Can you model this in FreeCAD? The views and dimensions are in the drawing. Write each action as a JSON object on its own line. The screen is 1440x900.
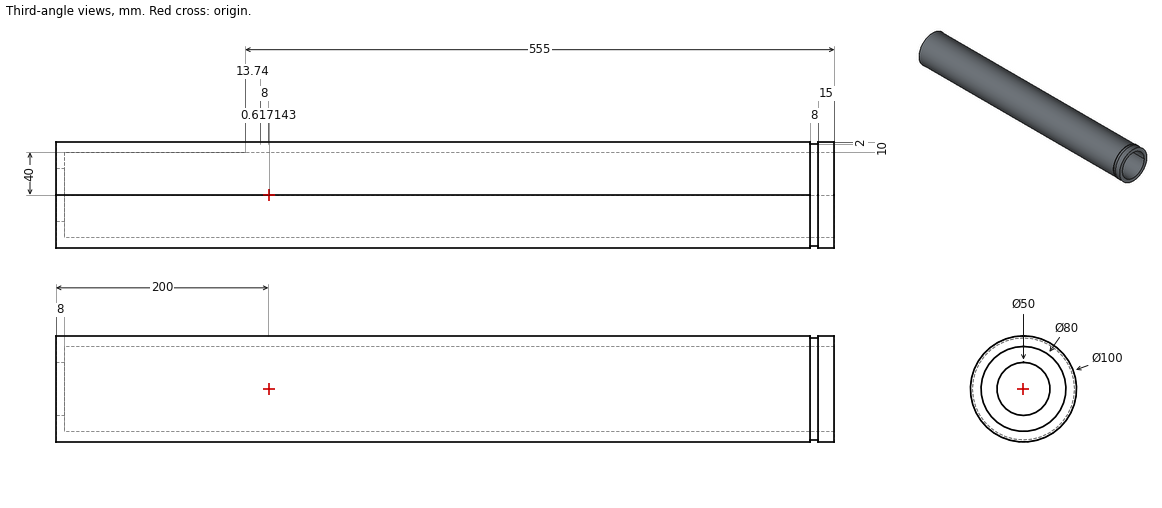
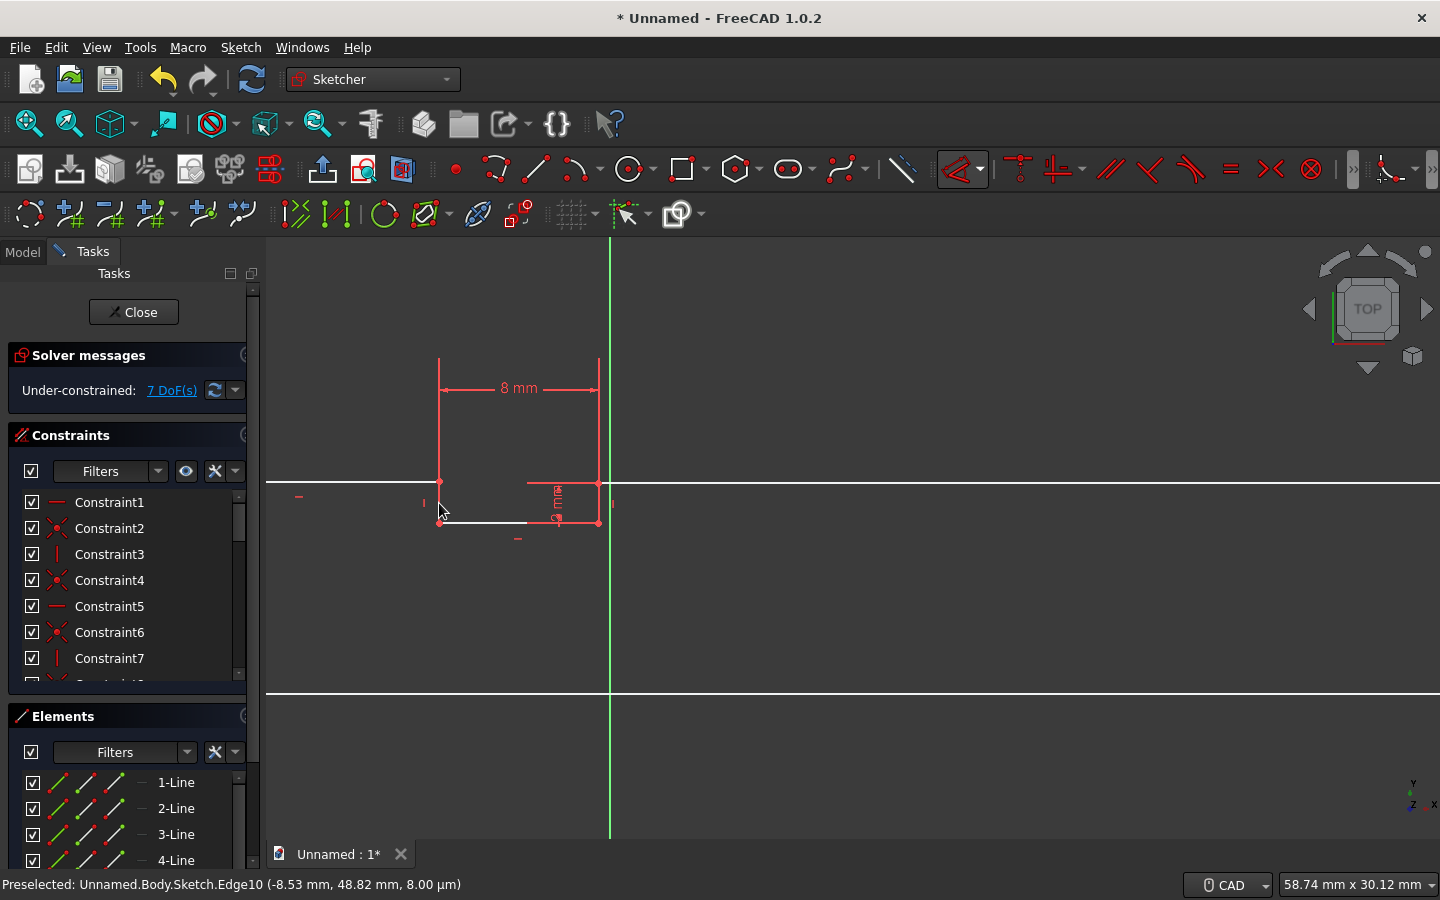
{"action": "key", "text": "i"}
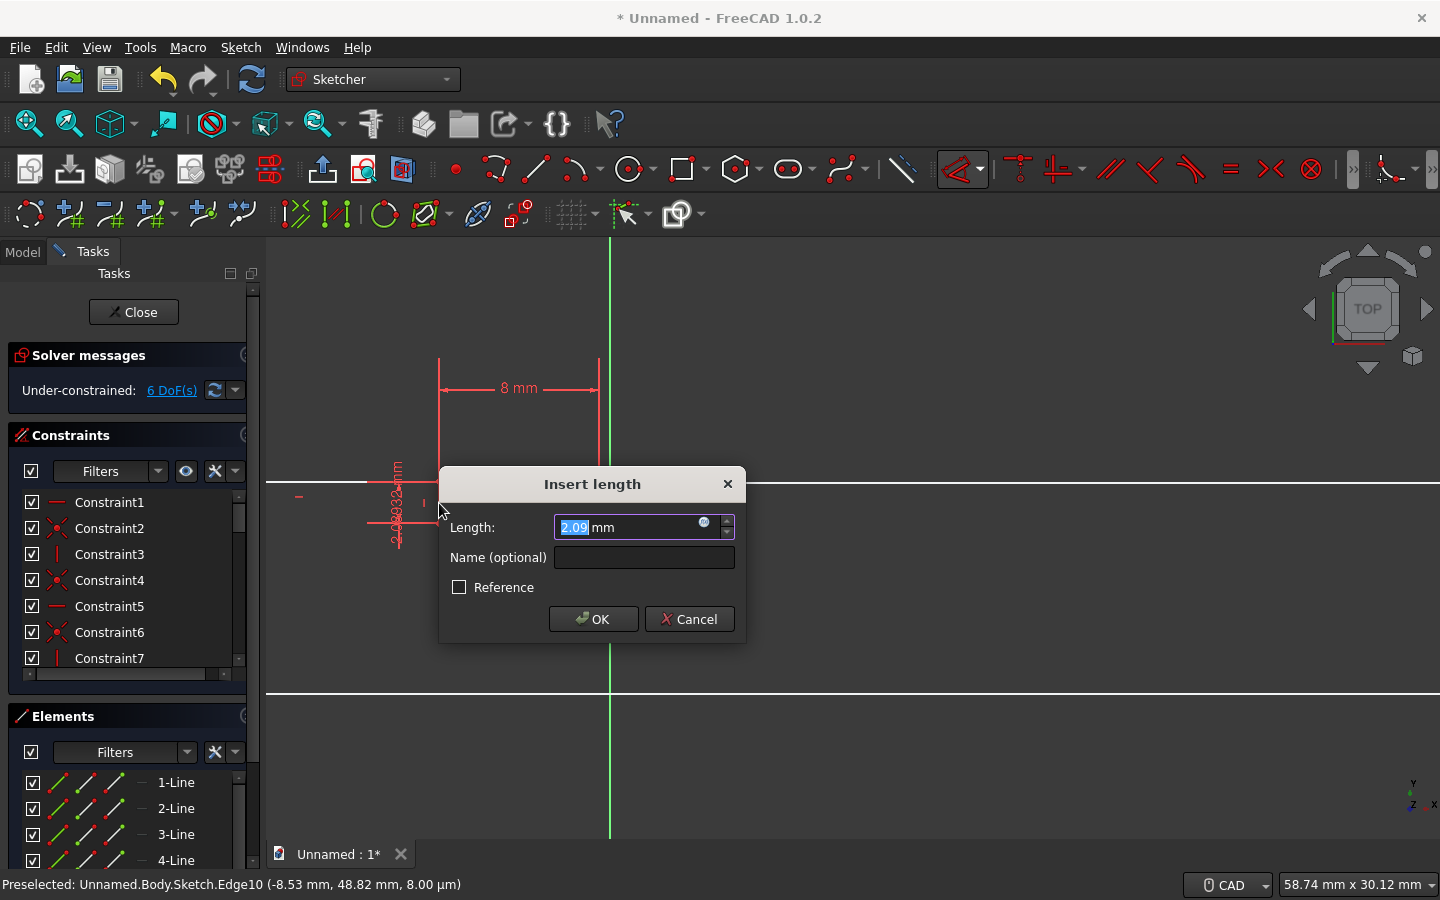
{"action": "type", "text": "2"}
{"action": "key", "text": "Return"}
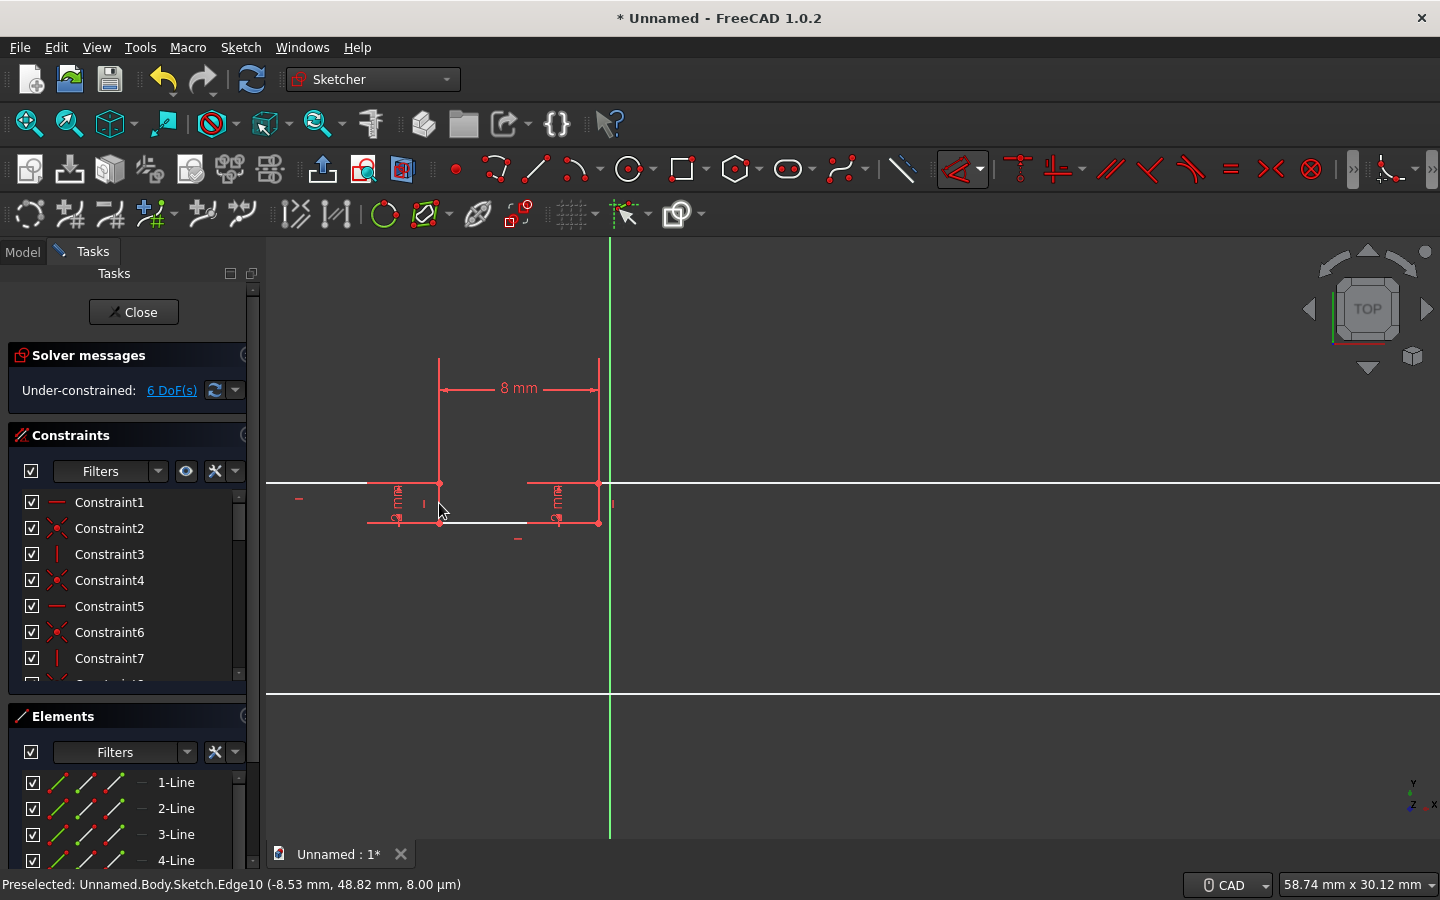
{"action": "scroll", "coordinate": [466, 509], "scroll_direction": "down", "scroll_amount": 14}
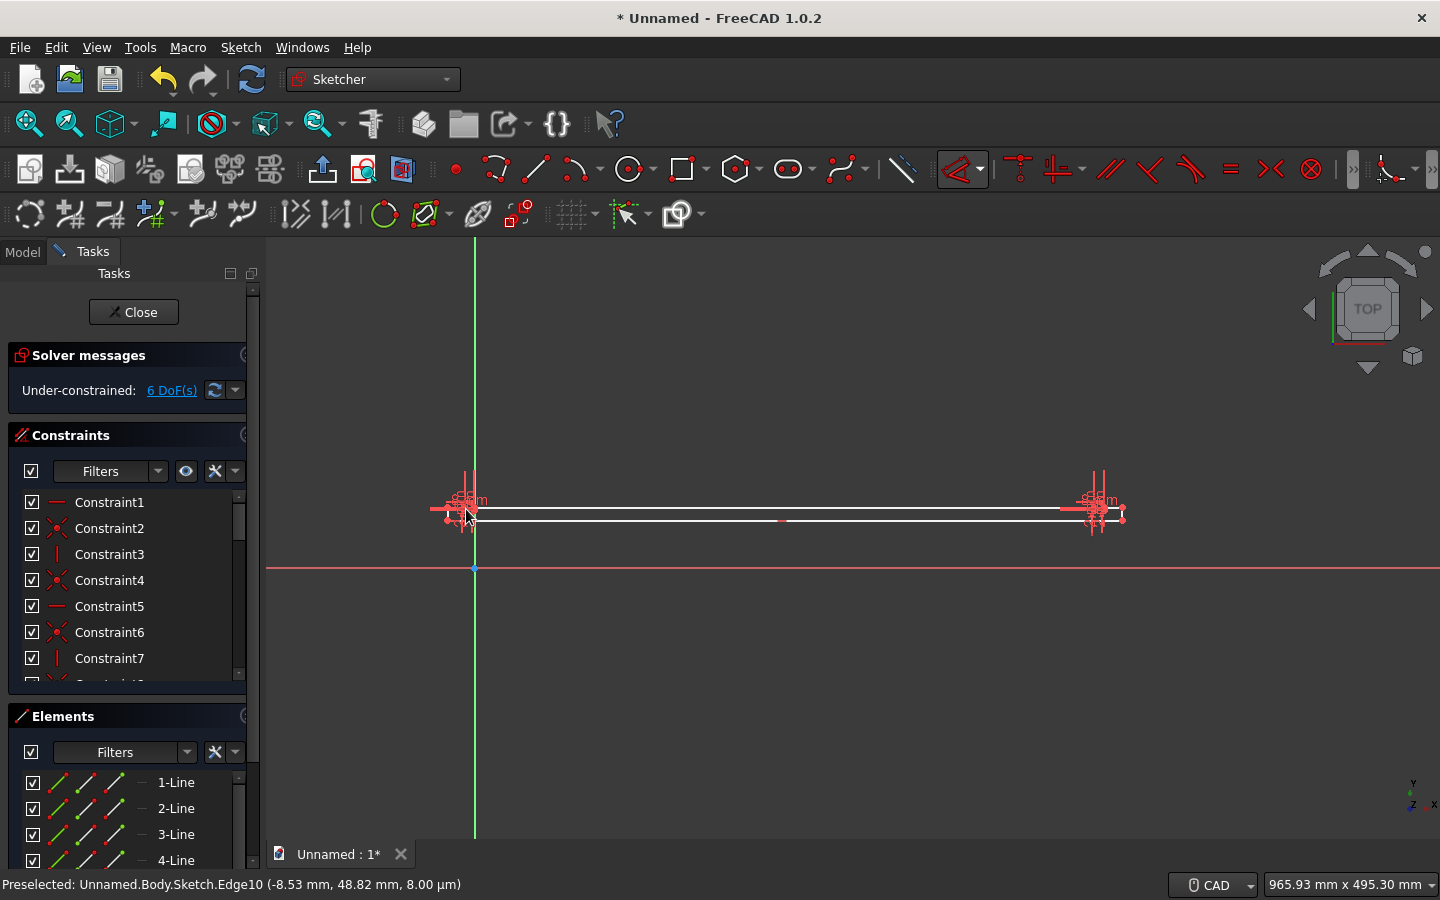
{"action": "scroll", "coordinate": [1122, 517], "scroll_direction": "up", "scroll_amount": 7}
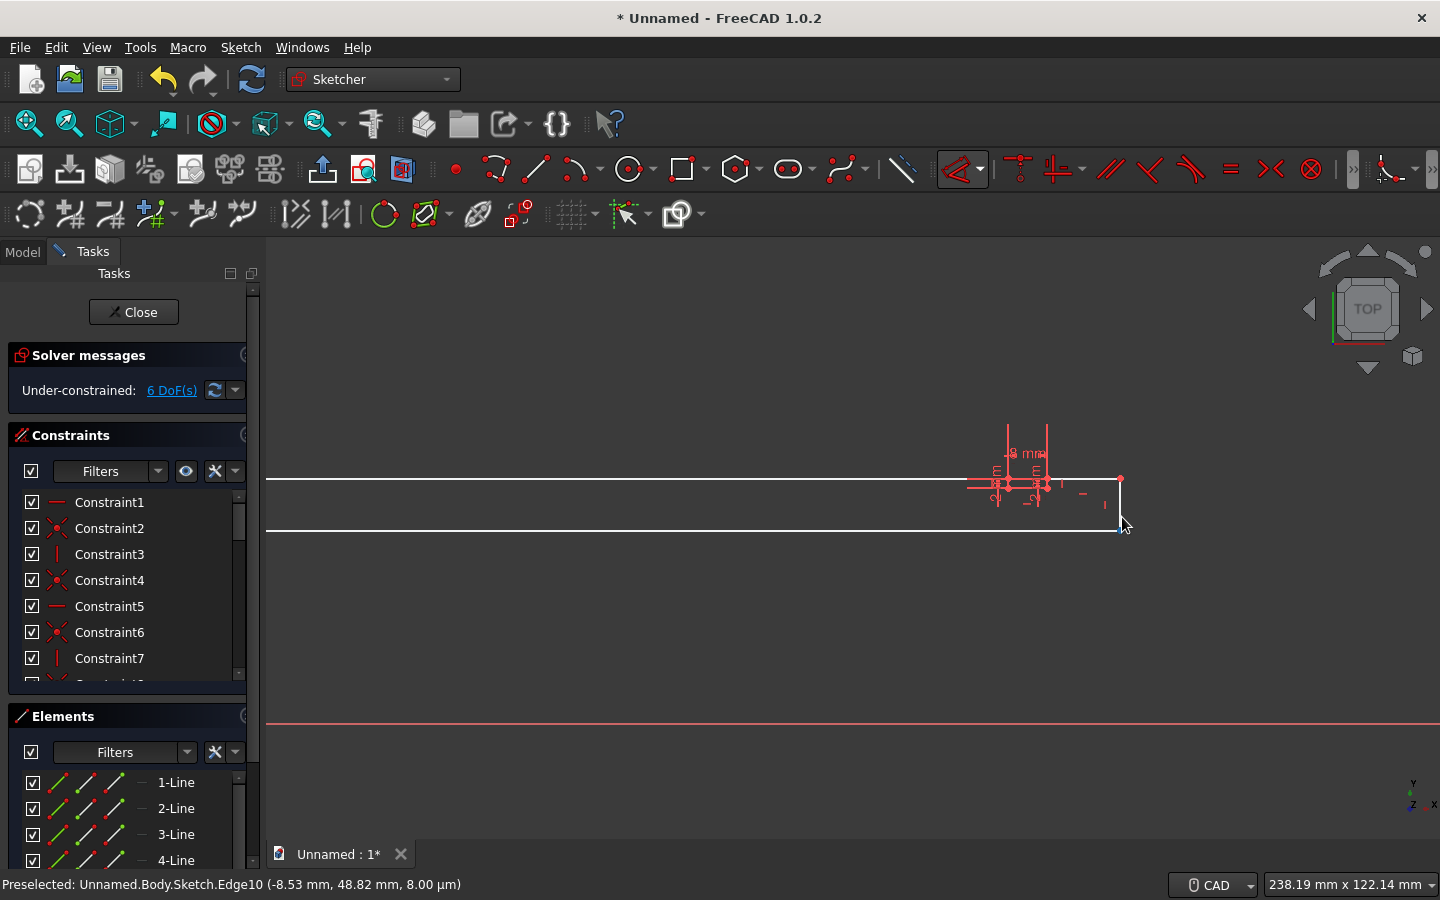
{"action": "left_click", "coordinate": [1120, 515]}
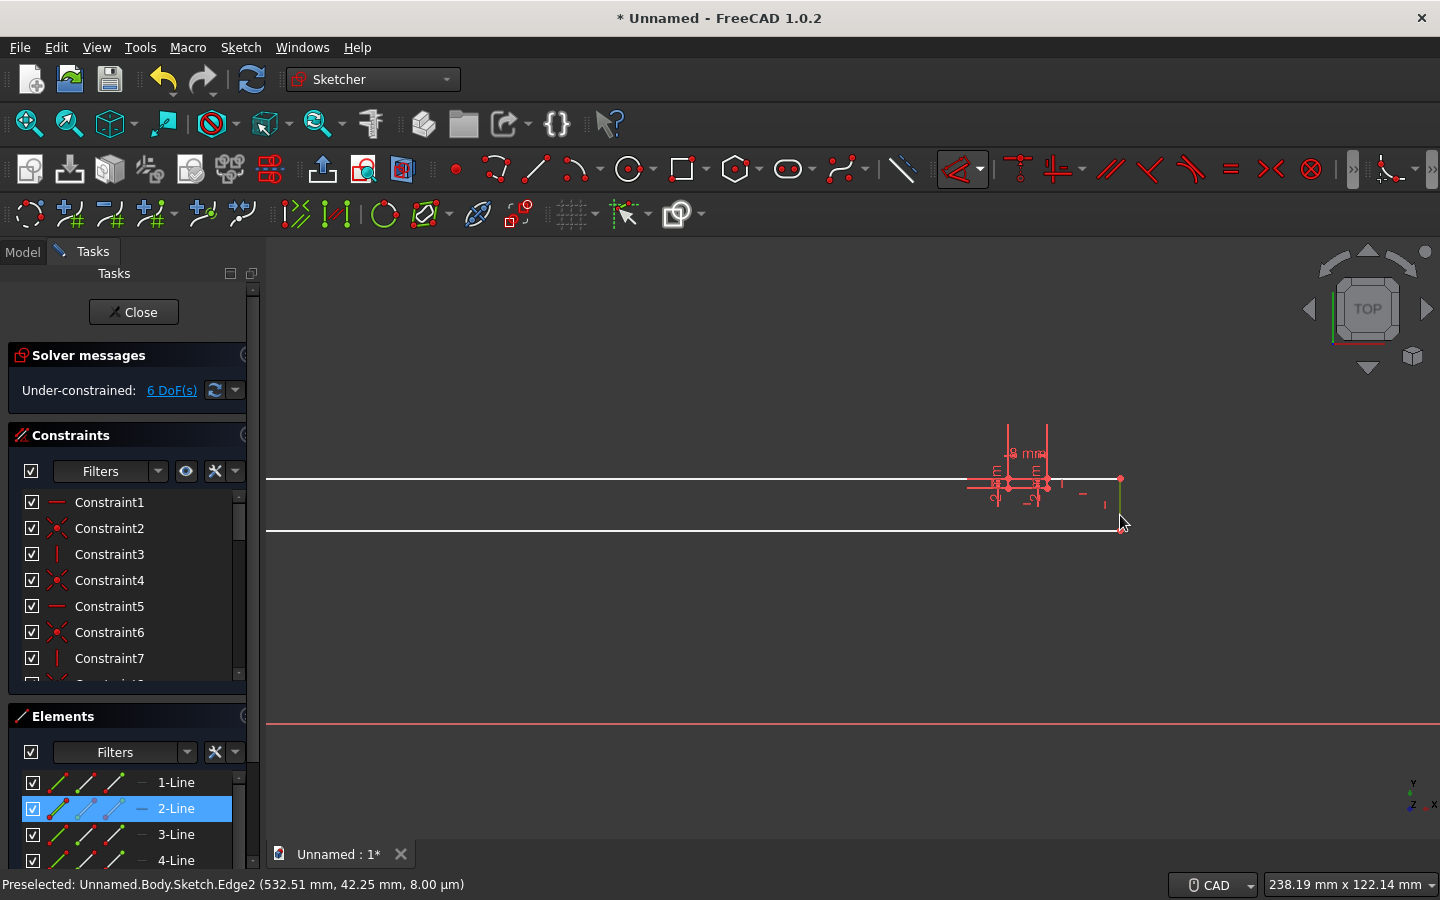
{"action": "key", "text": "i"}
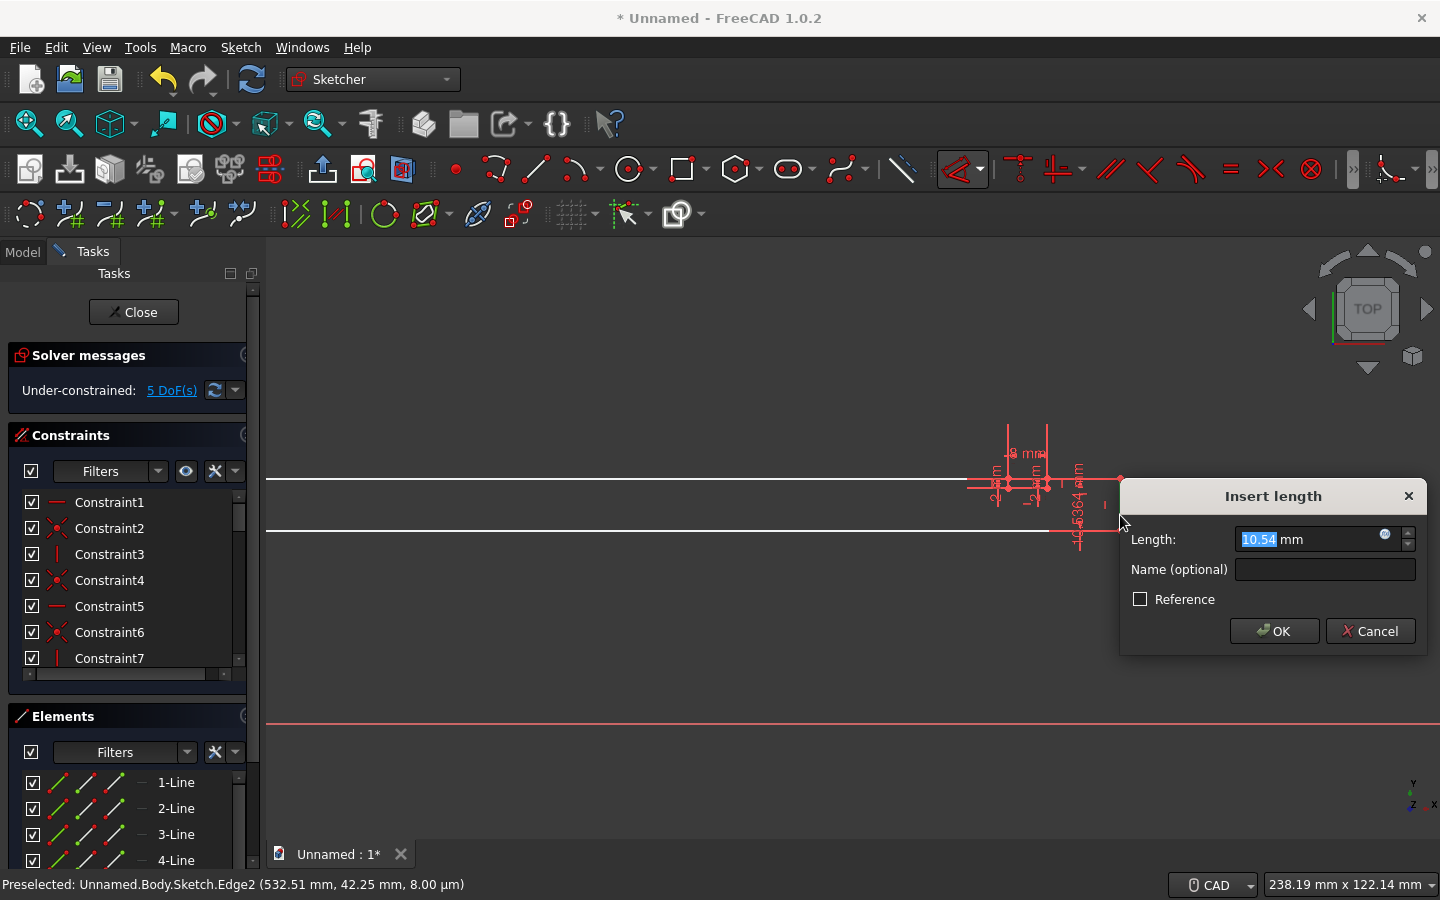
{"action": "type", "text": "10"}
{"action": "key", "text": "Return"}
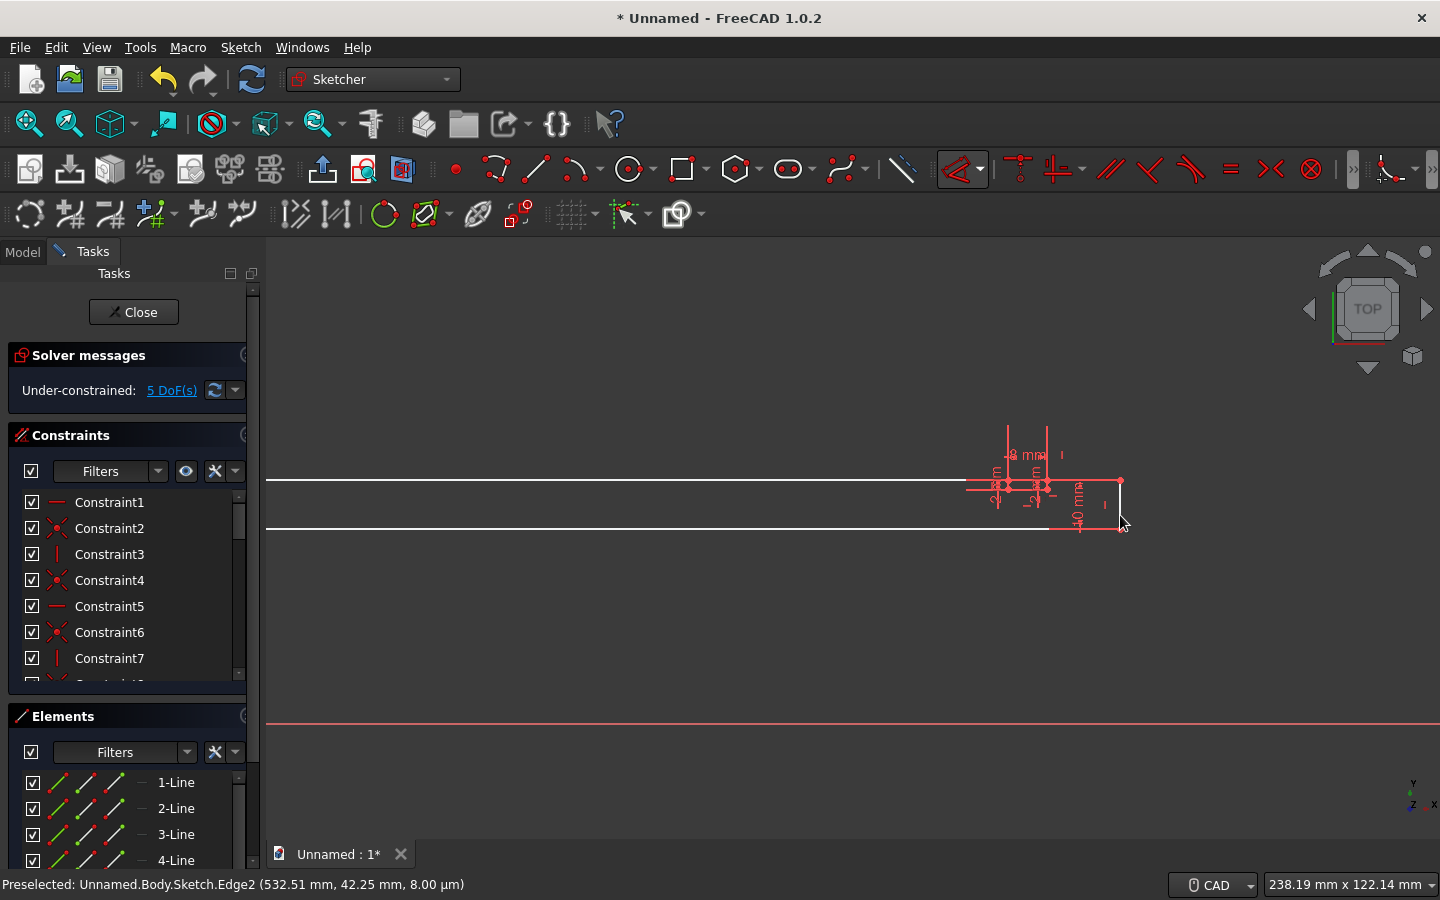
{"action": "left_click", "coordinate": [1098, 480]}